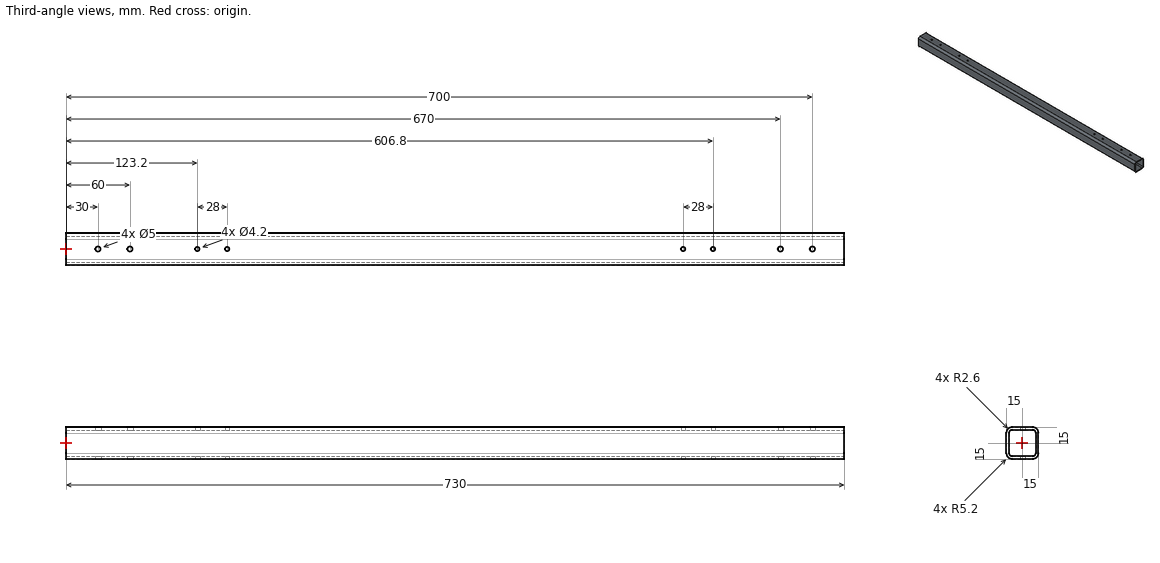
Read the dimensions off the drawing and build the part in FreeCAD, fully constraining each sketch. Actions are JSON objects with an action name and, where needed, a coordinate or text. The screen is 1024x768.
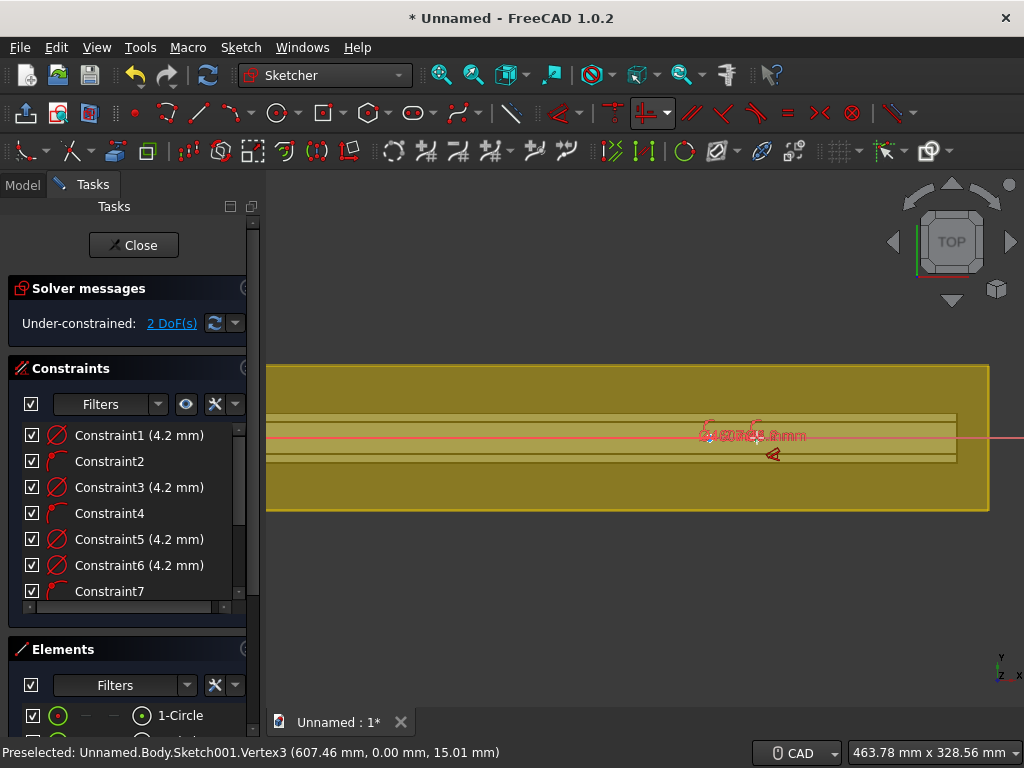
{"action": "left_click", "coordinate": [710, 438]}
{"action": "left_click", "coordinate": [733, 472]}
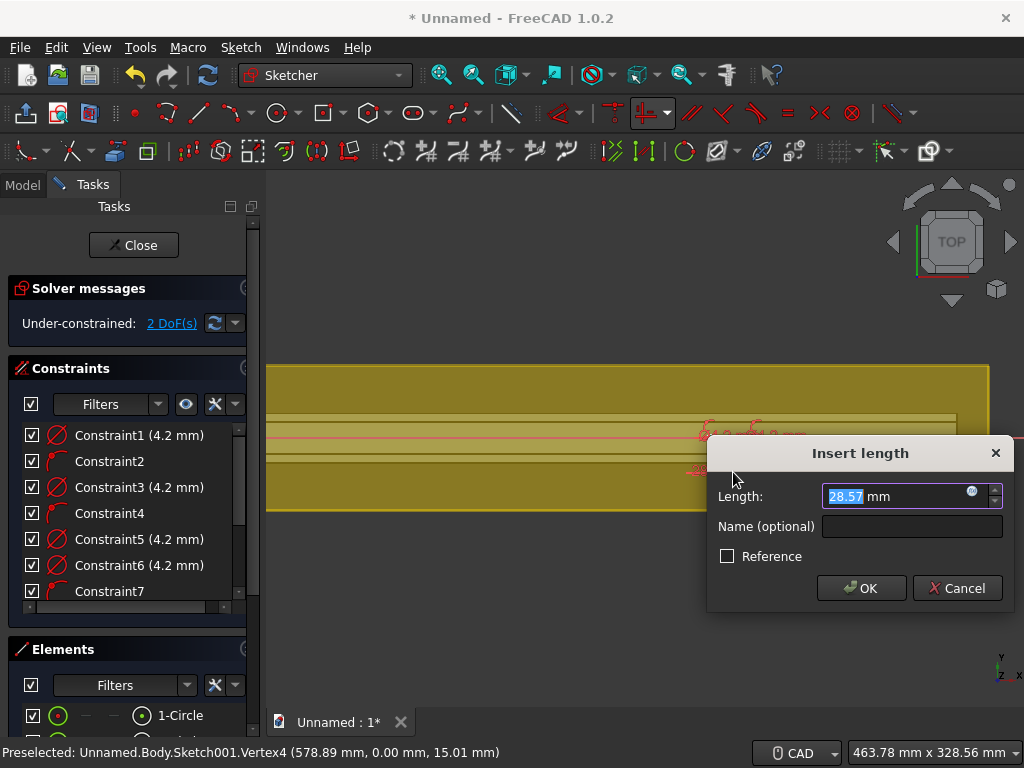
{"action": "type", "text": "28"}
{"action": "key", "text": "Return"}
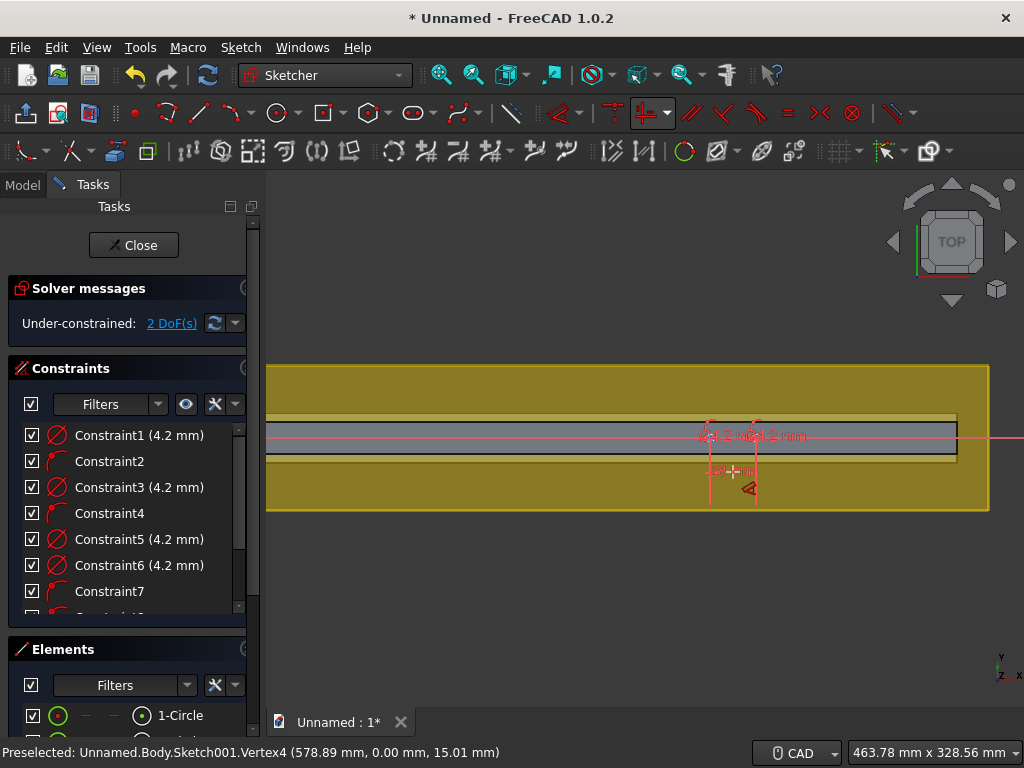
{"action": "scroll", "coordinate": [760, 439], "scroll_direction": "down", "scroll_amount": 5}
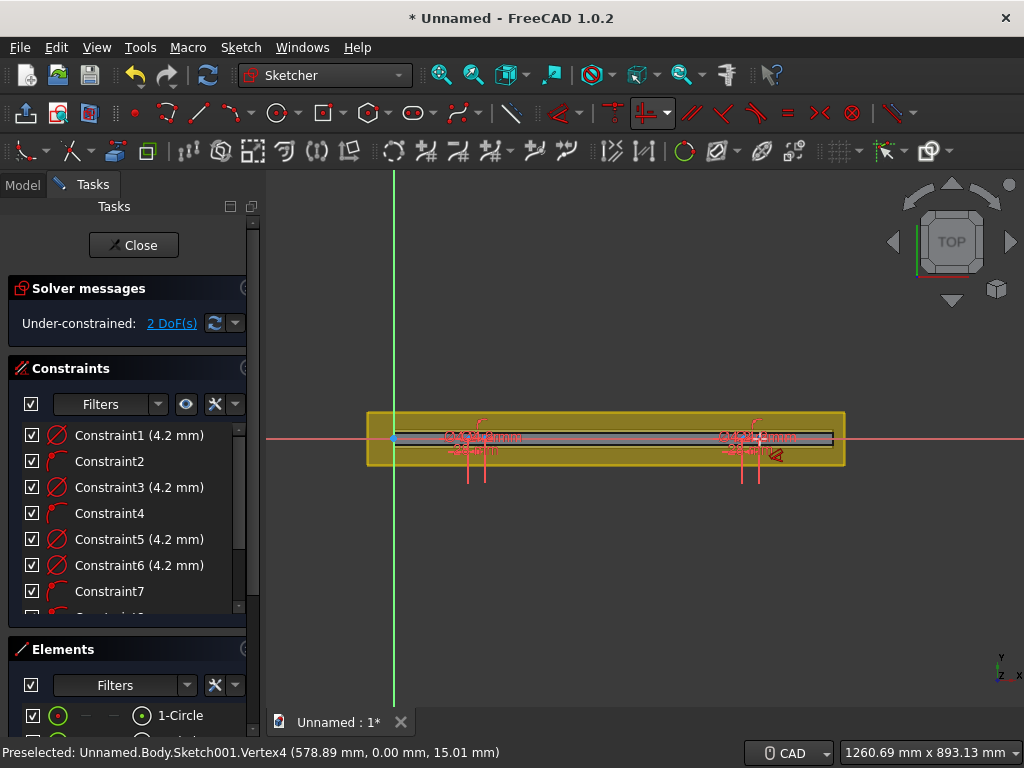
{"action": "left_click", "coordinate": [468, 439]}
{"action": "left_click", "coordinate": [431, 473]}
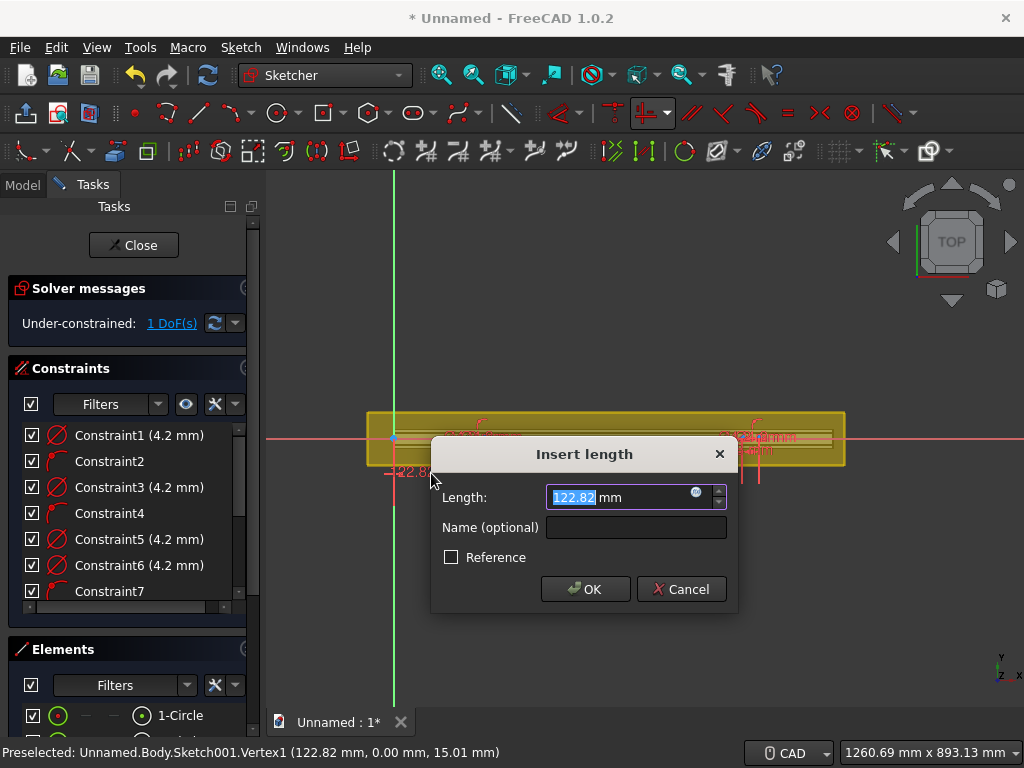
{"action": "type", "text": "123.2"}
{"action": "key", "text": "Return"}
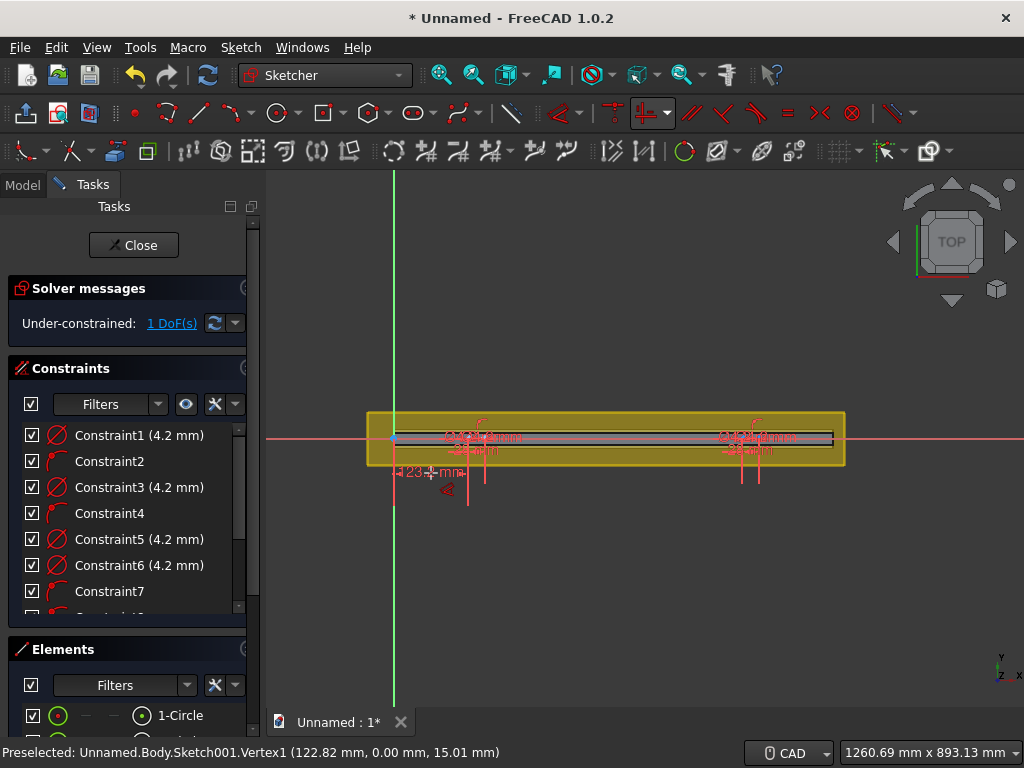
{"action": "left_click", "coordinate": [759, 439]}
{"action": "left_click", "coordinate": [576, 473]}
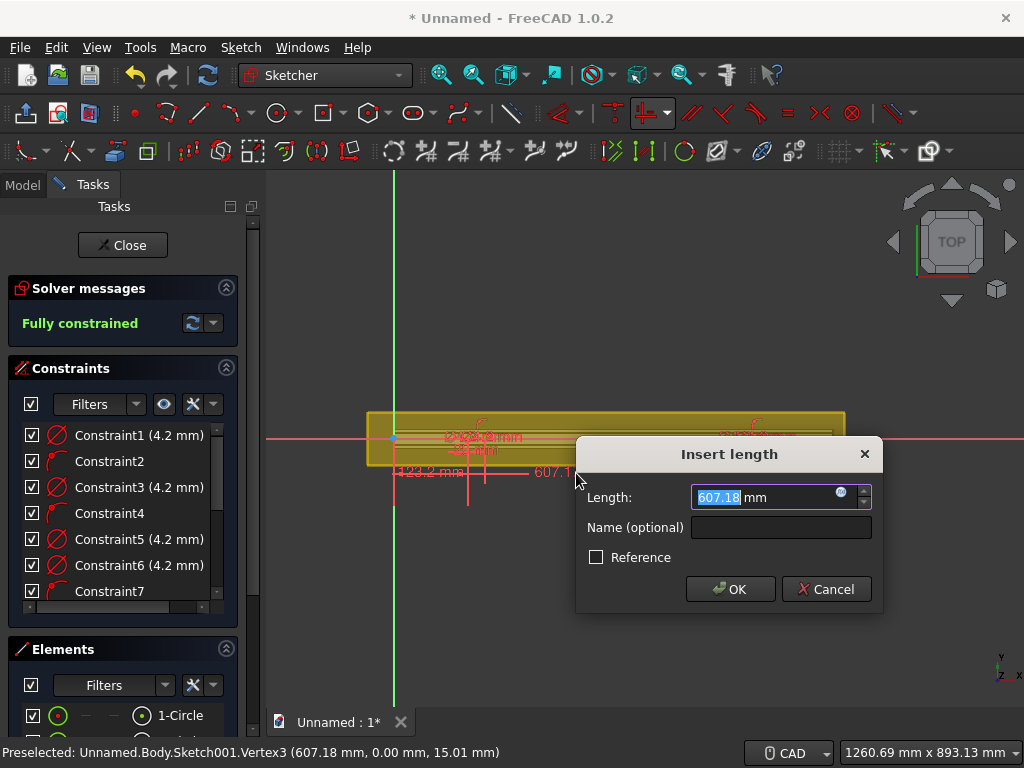
{"action": "type", "text": "606.8"}
{"action": "key", "text": "Return"}
{"action": "key", "text": "Escape"}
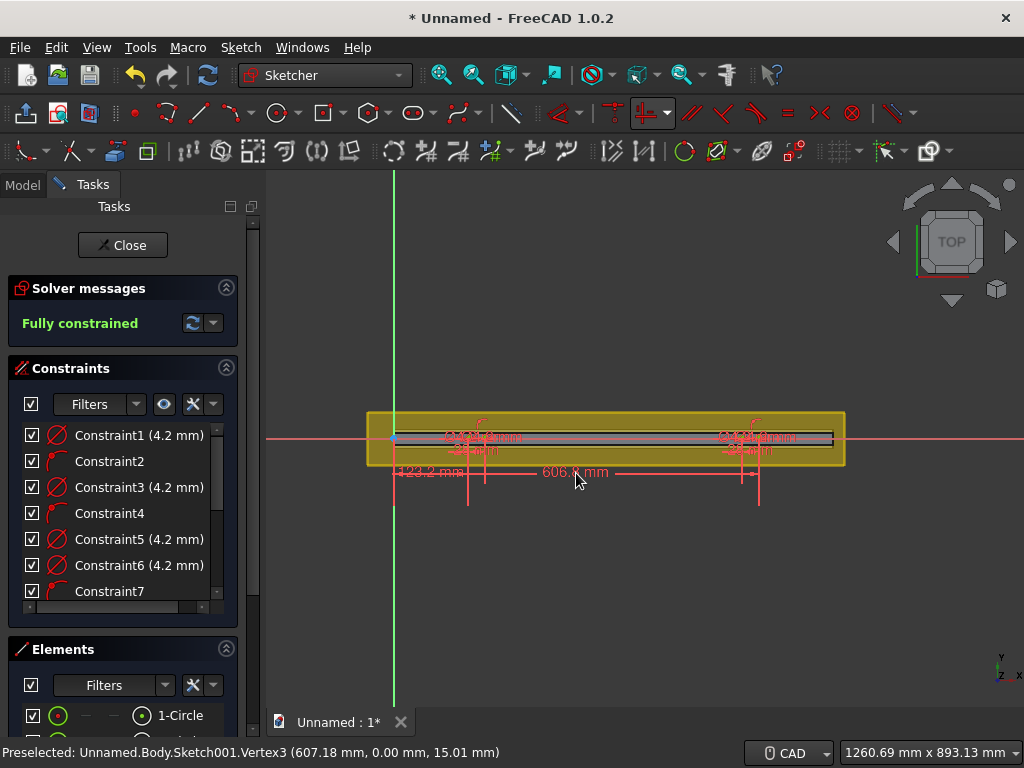
{"action": "left_click", "coordinate": [123, 245]}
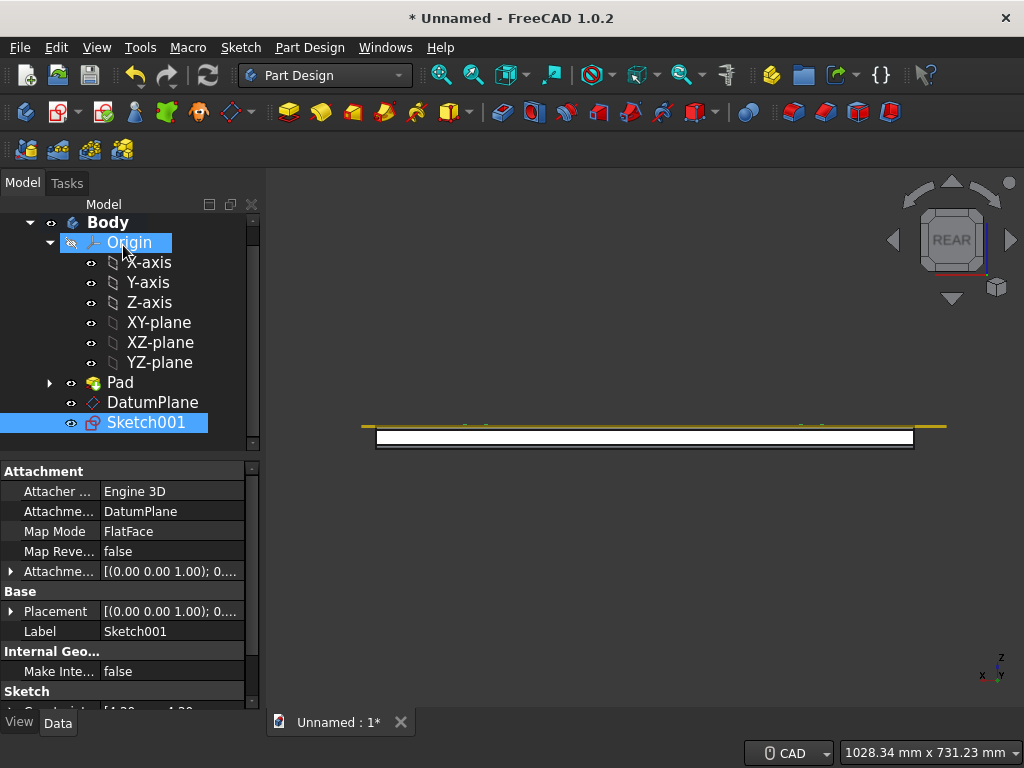
{"action": "left_click", "coordinate": [504, 112]}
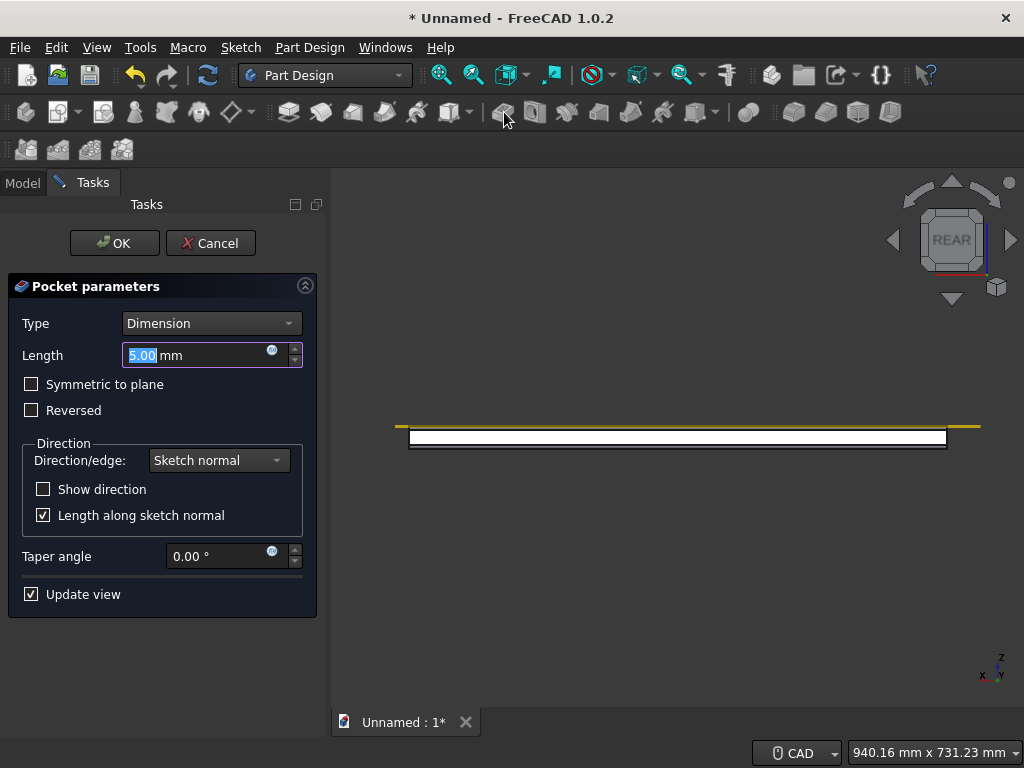
{"action": "left_click", "coordinate": [212, 324]}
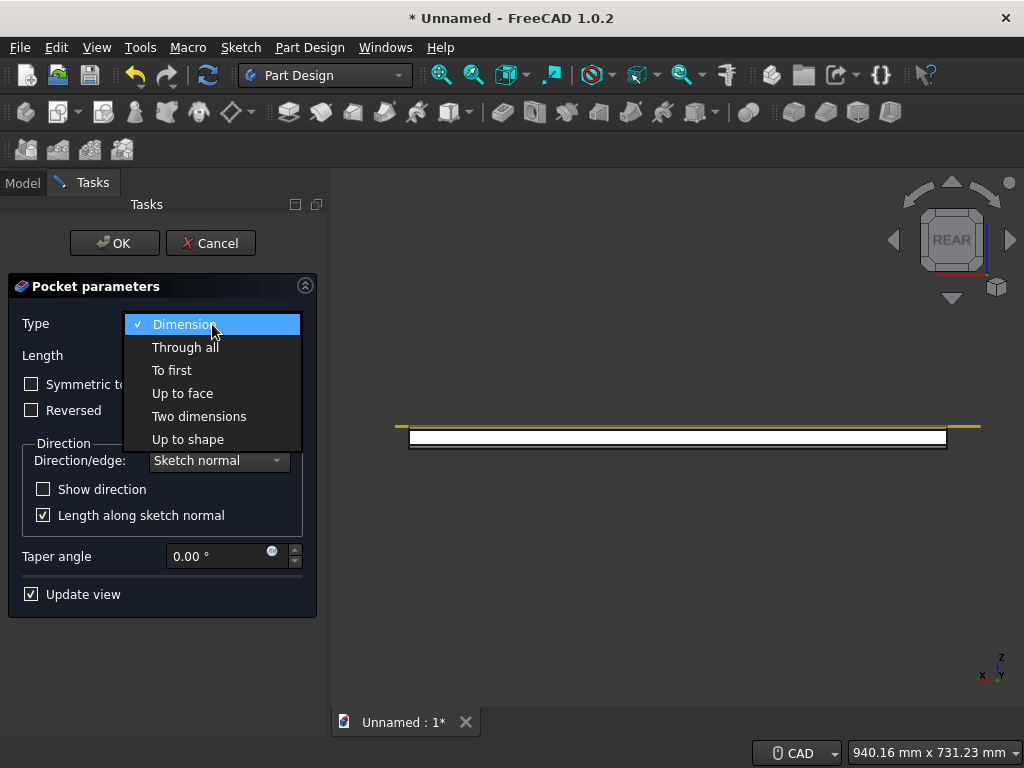
{"action": "left_click", "coordinate": [212, 348]}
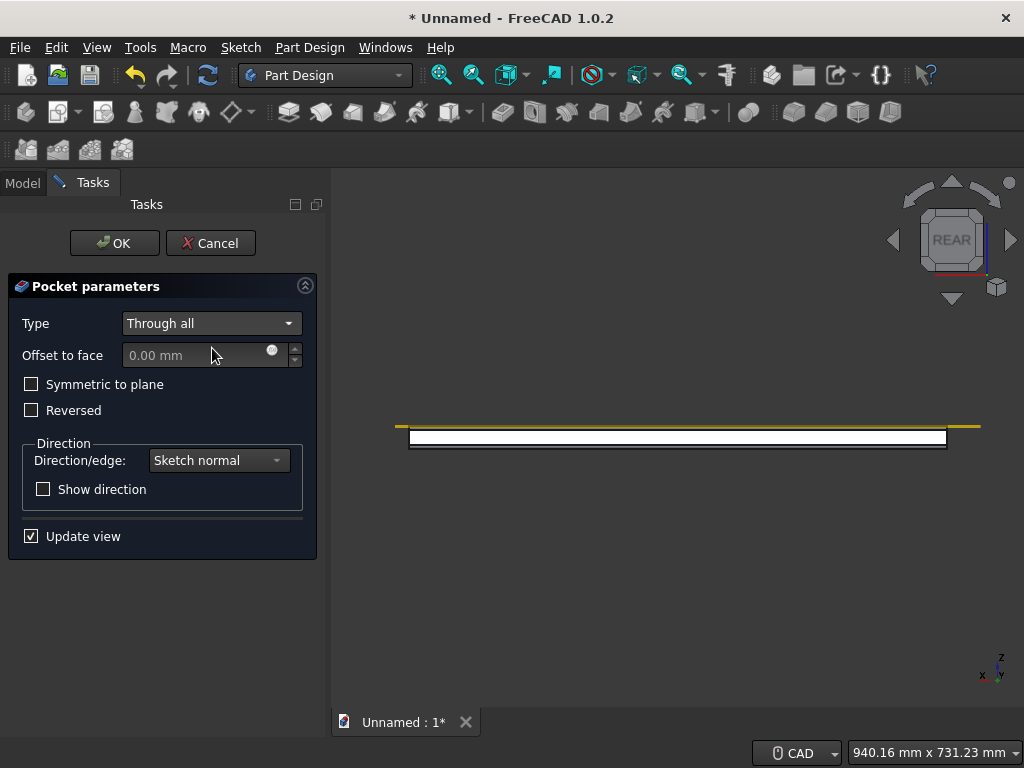
{"action": "left_click", "coordinate": [115, 243]}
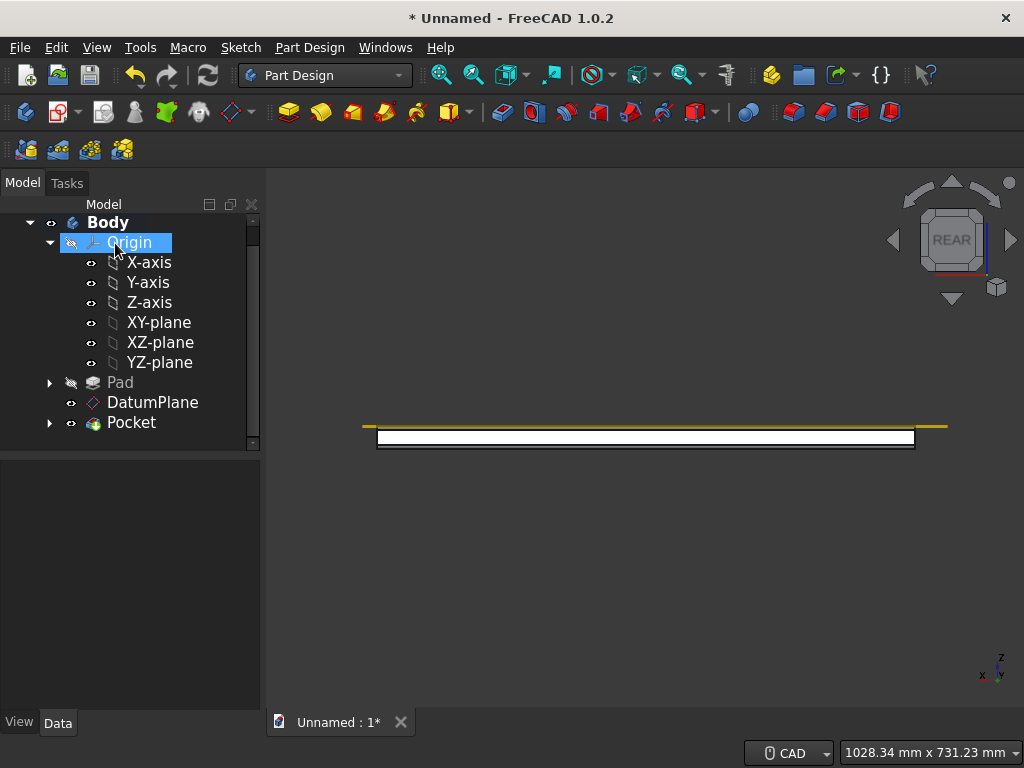
{"action": "left_click", "coordinate": [116, 403]}
{"action": "key", "text": "space"}